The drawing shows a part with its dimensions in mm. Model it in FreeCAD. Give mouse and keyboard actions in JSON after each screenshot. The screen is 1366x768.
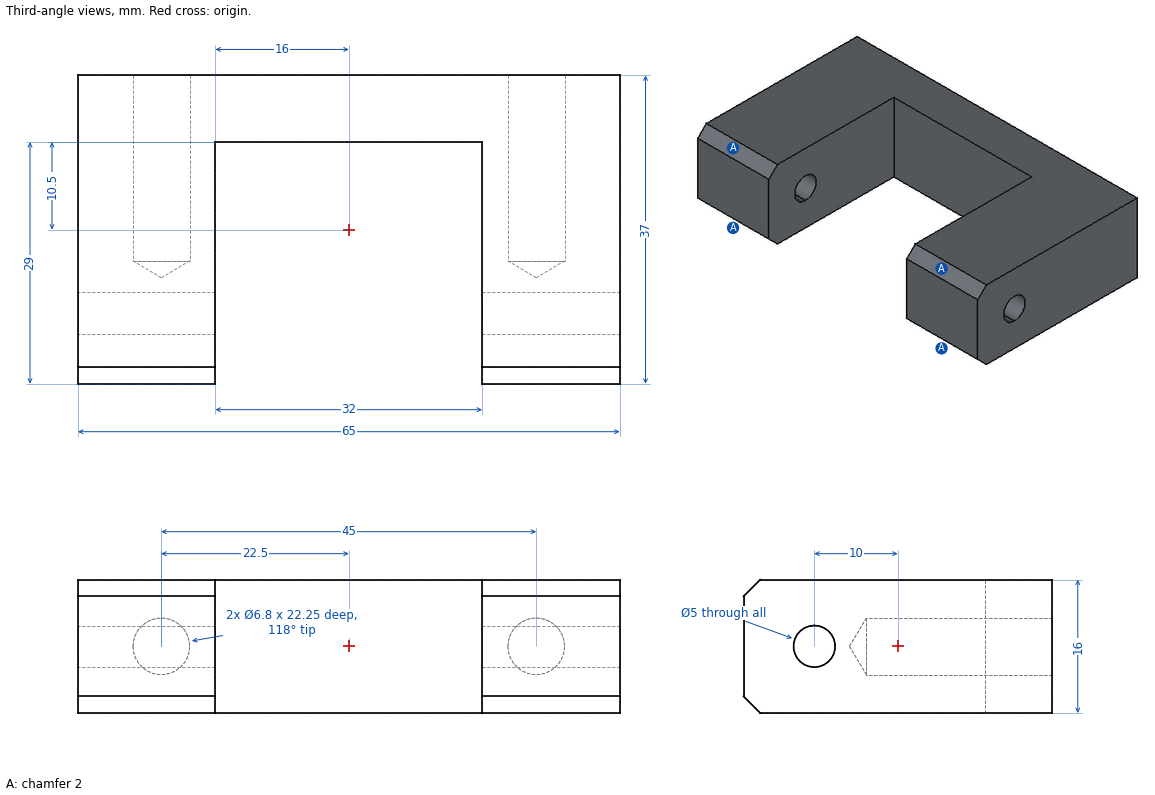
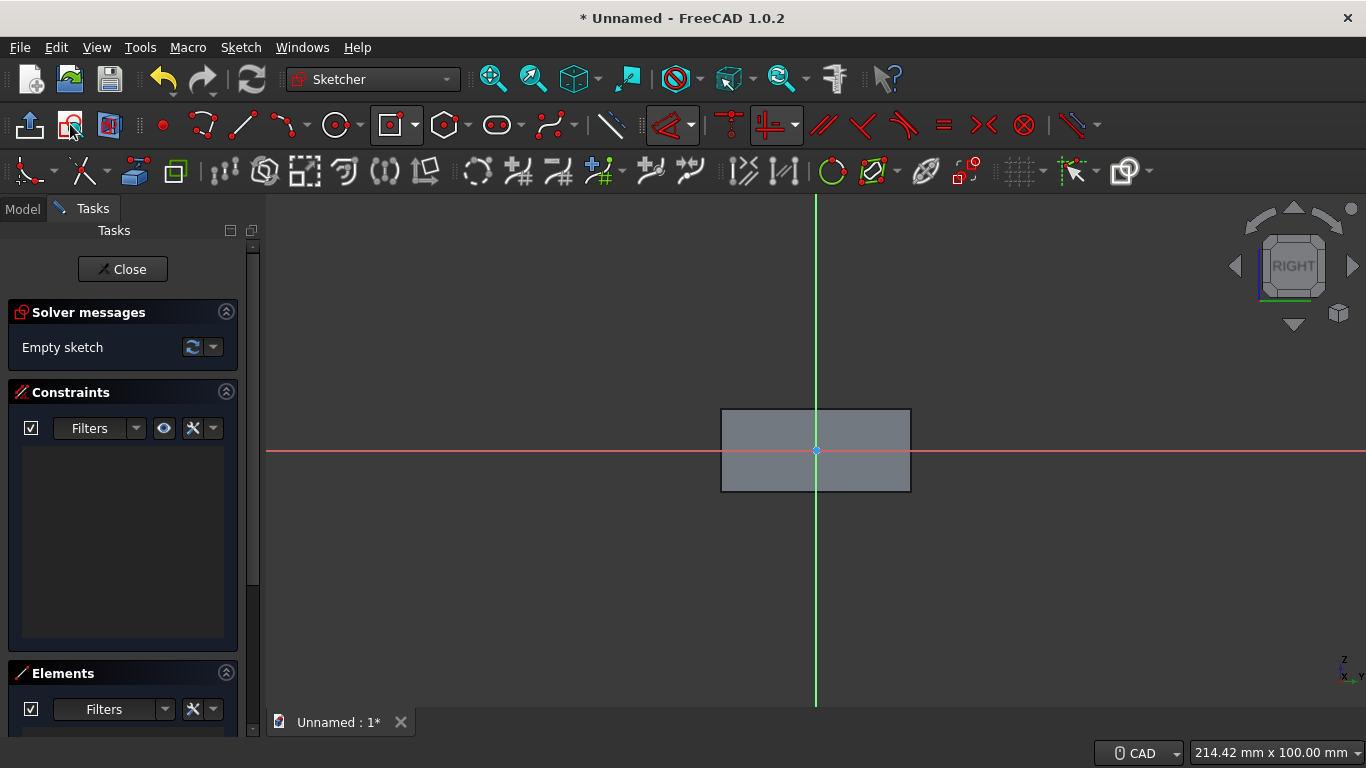
{"action": "scroll", "coordinate": [766, 450], "scroll_direction": "up", "scroll_amount": 13}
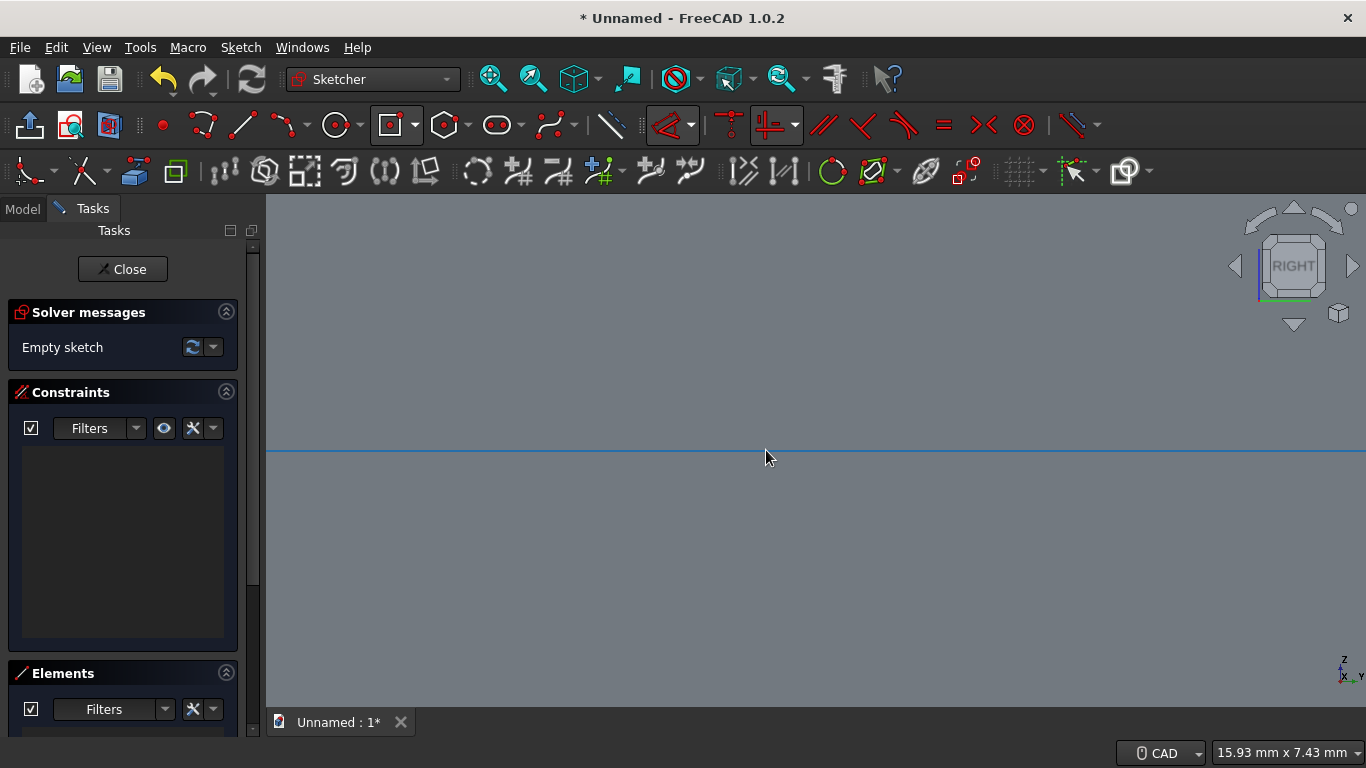
{"action": "left_click", "coordinate": [336, 126]}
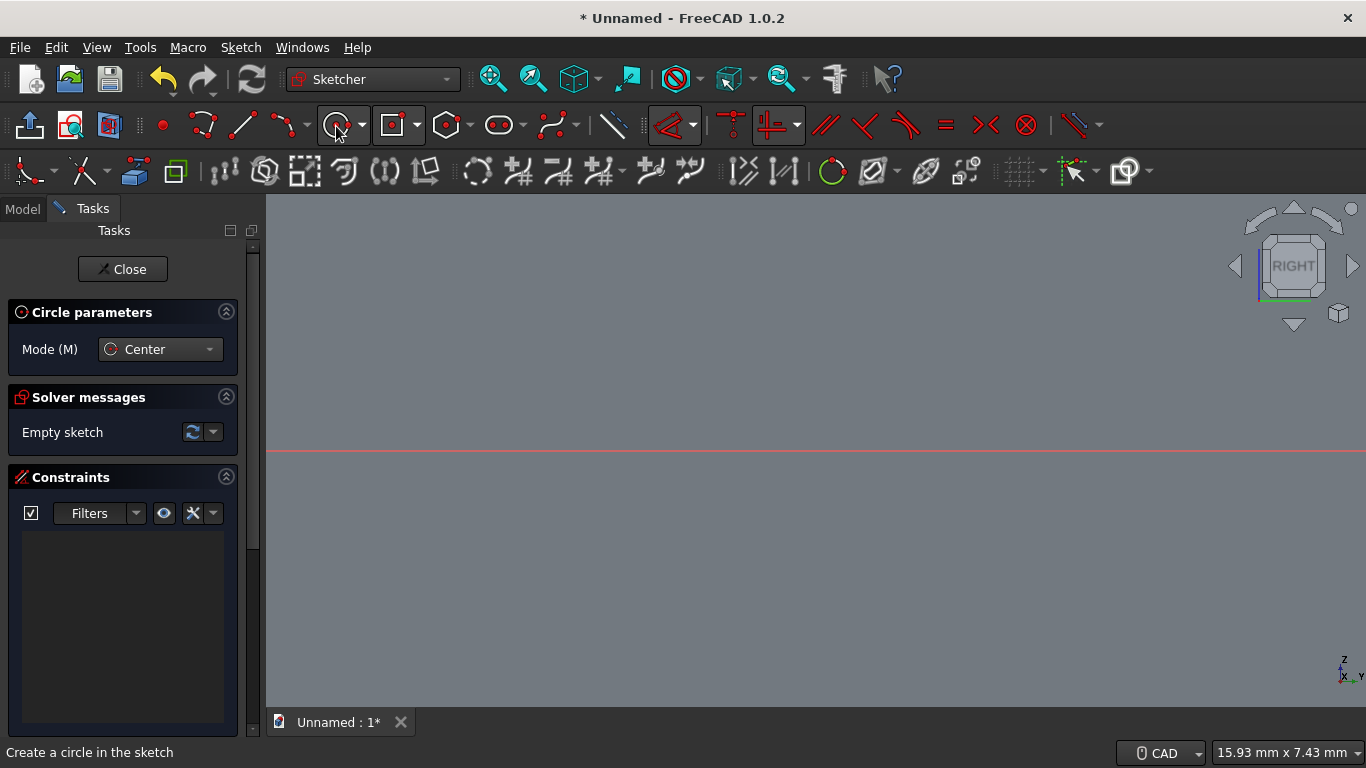
{"action": "left_click", "coordinate": [743, 450]}
{"action": "left_click", "coordinate": [865, 328]}
{"action": "key", "text": "Escape"}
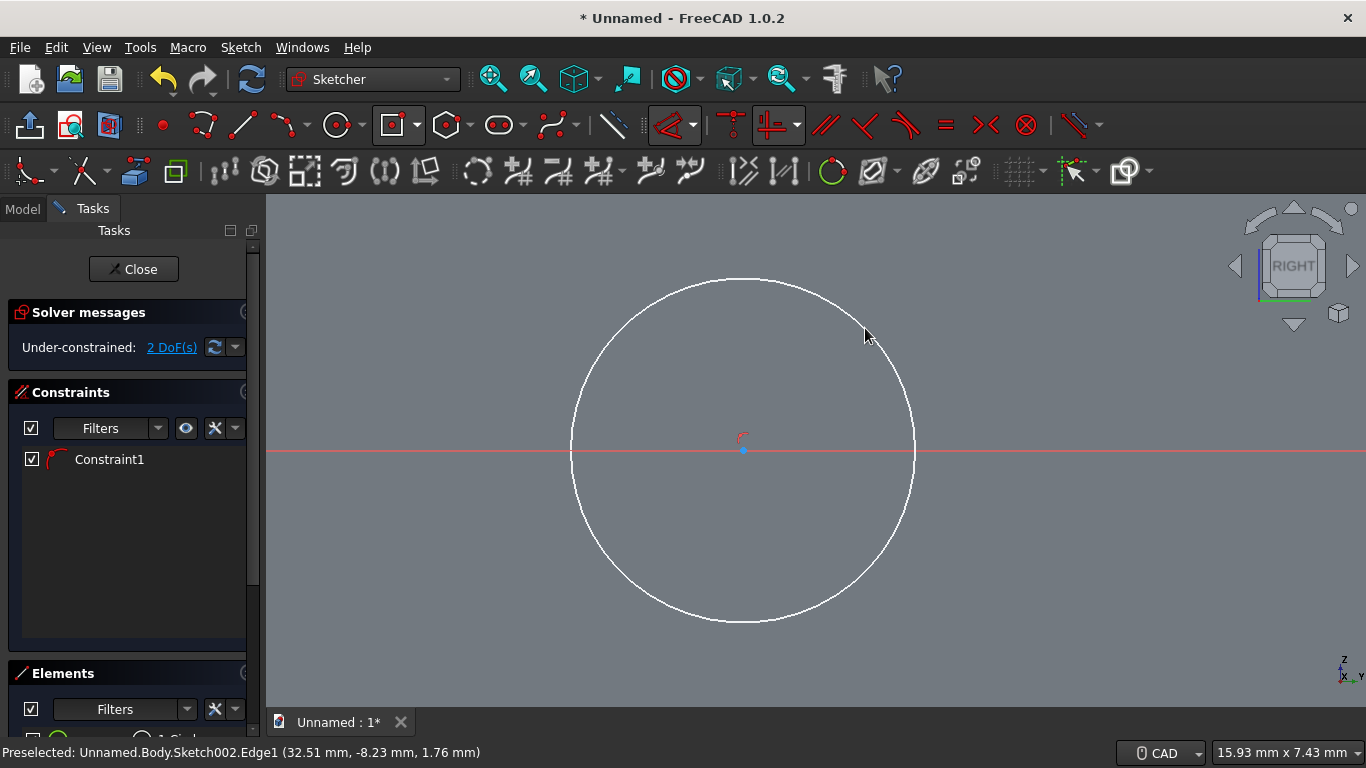
{"action": "left_click", "coordinate": [864, 328]}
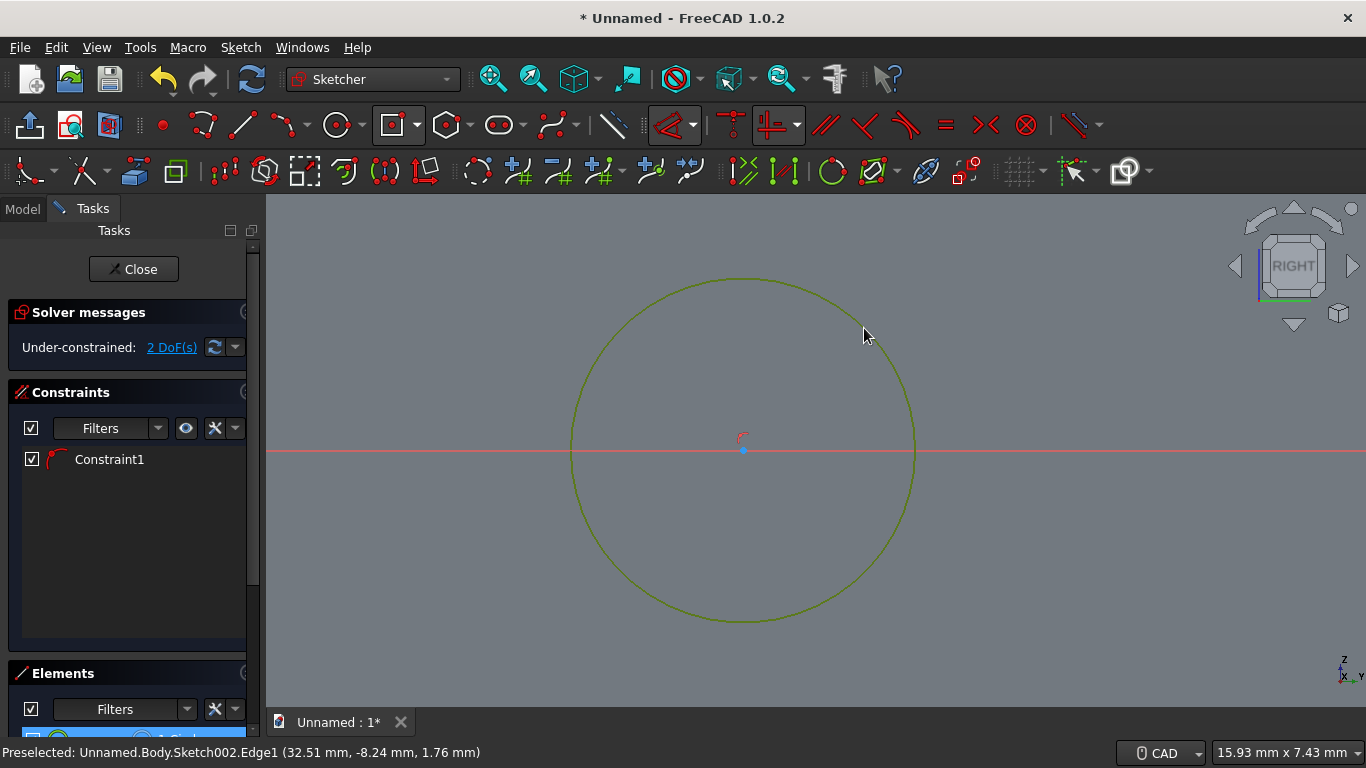
{"action": "key", "text": "k o"}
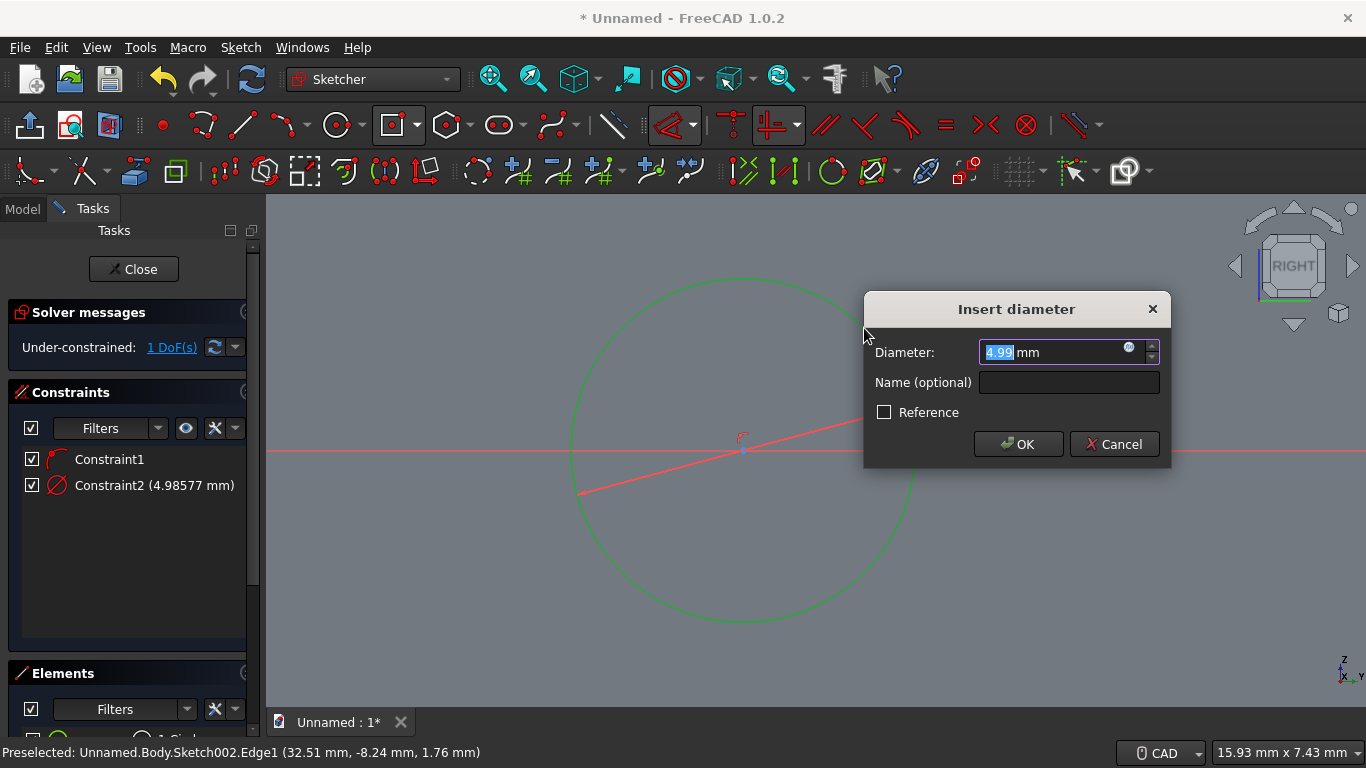
{"action": "type", "text": "5"}
{"action": "key", "text": "Return"}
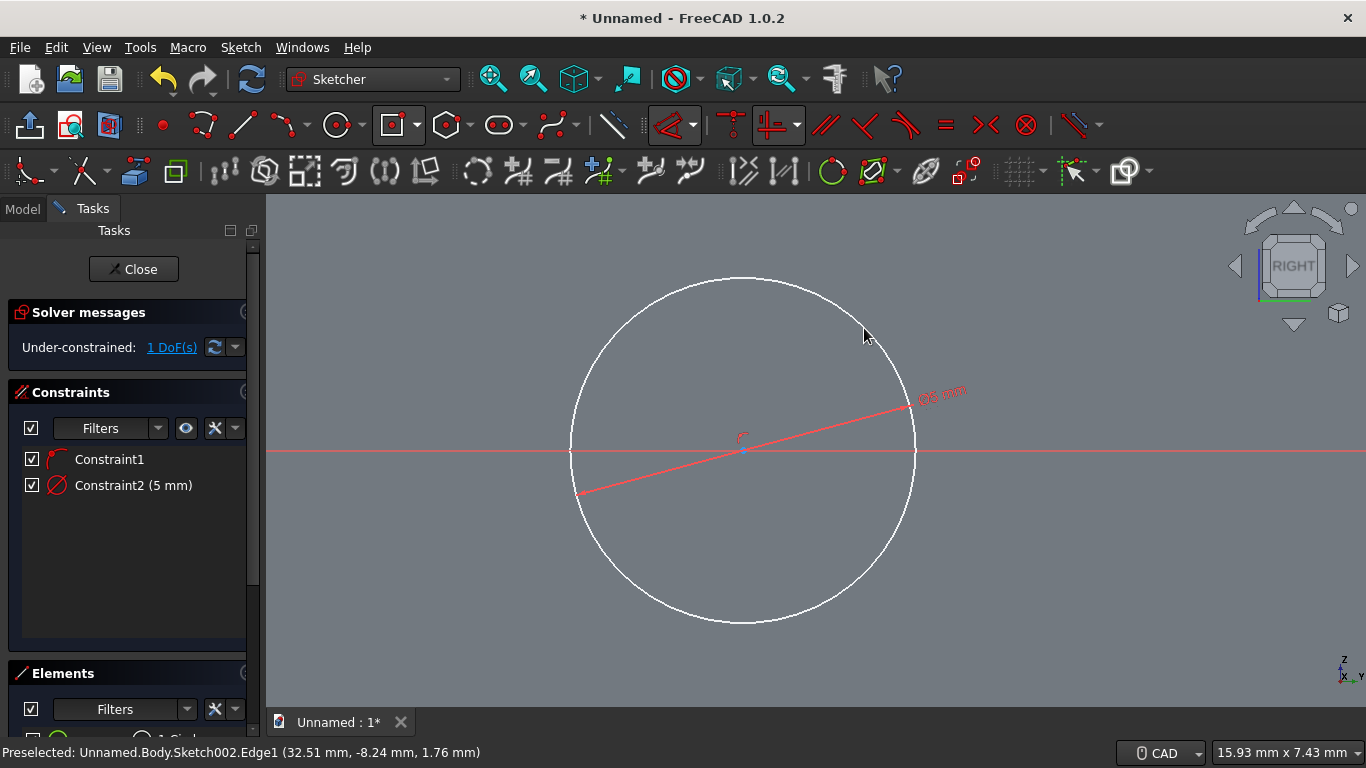
{"action": "left_click", "coordinate": [743, 450]}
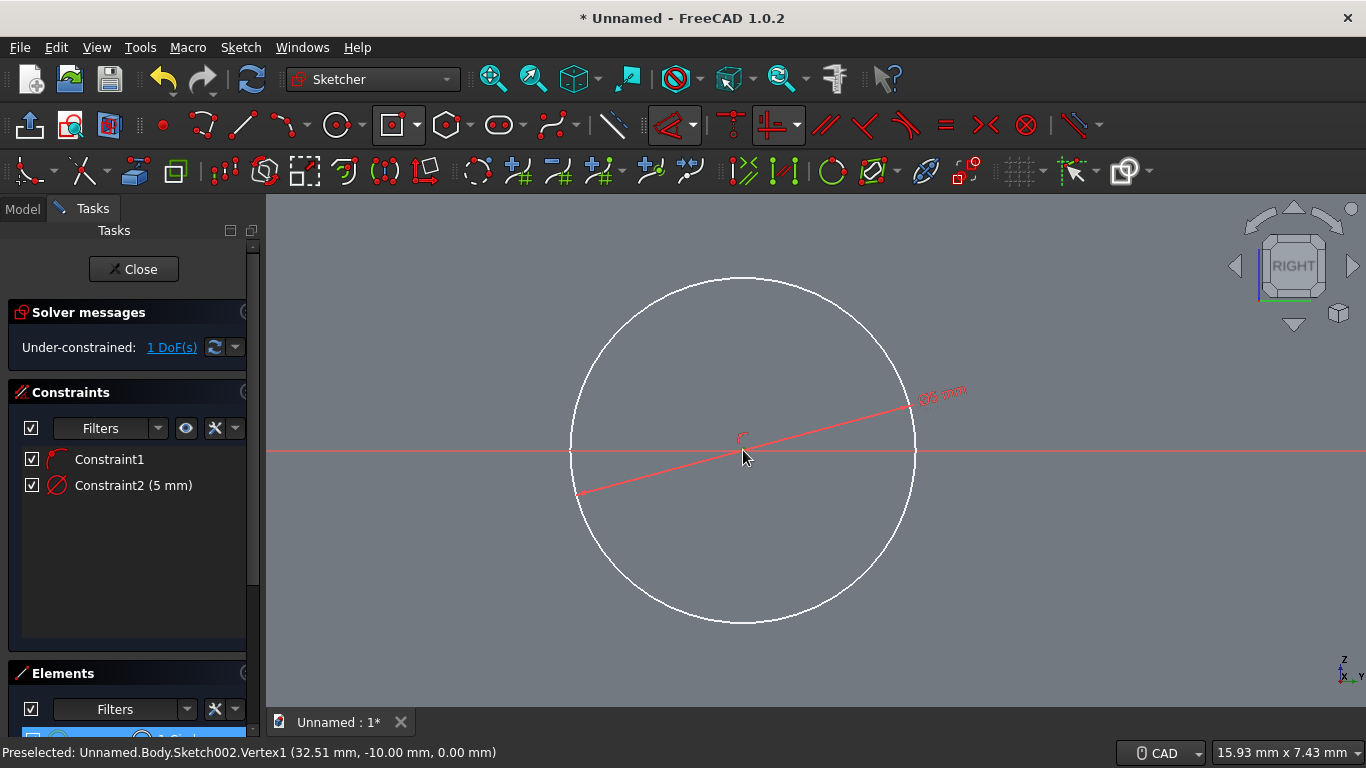
{"action": "left_click", "coordinate": [696, 126]}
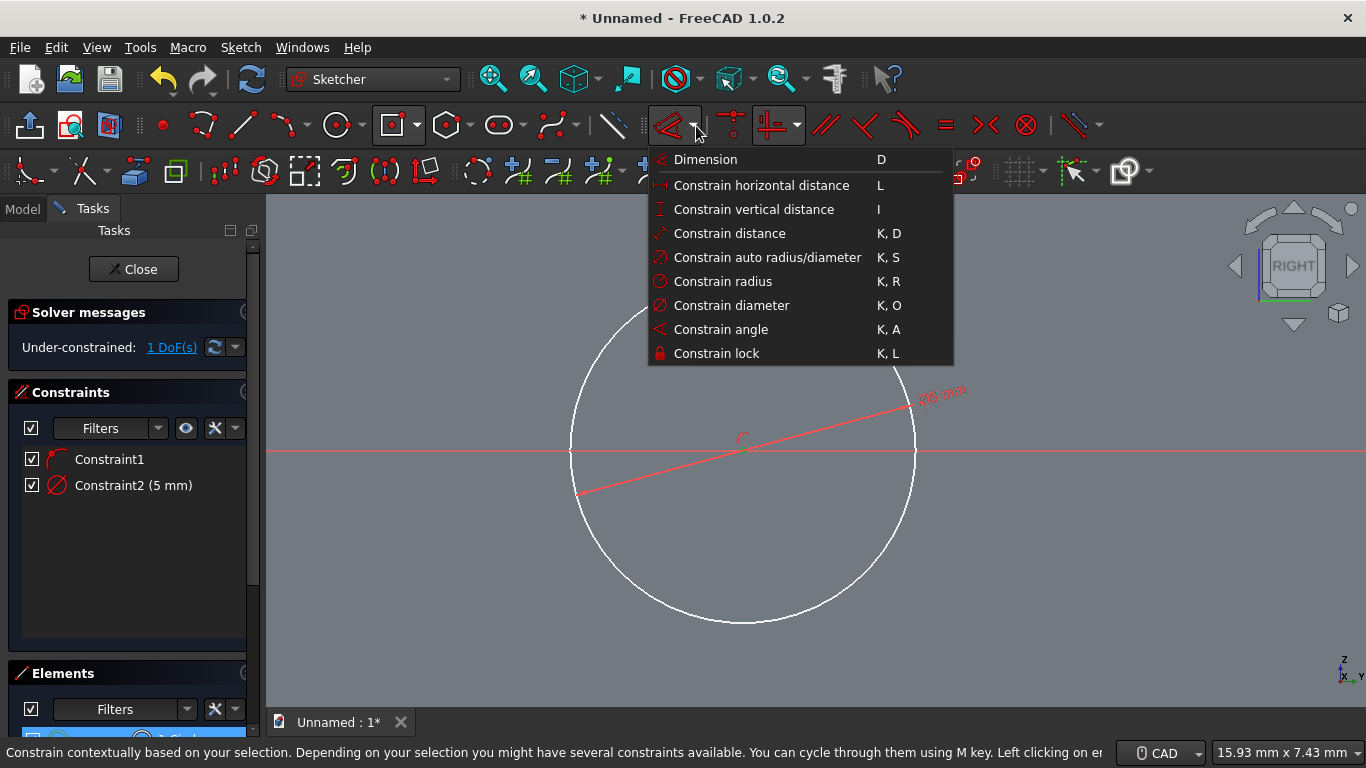
{"action": "left_click", "coordinate": [801, 185]}